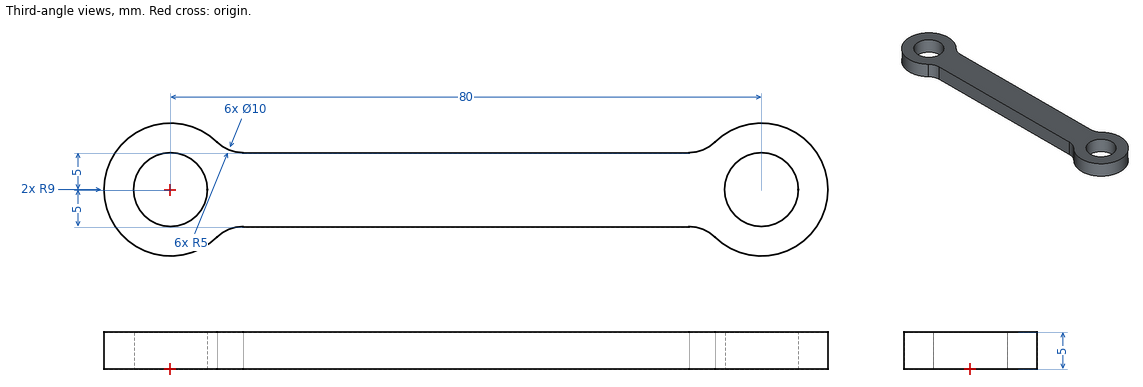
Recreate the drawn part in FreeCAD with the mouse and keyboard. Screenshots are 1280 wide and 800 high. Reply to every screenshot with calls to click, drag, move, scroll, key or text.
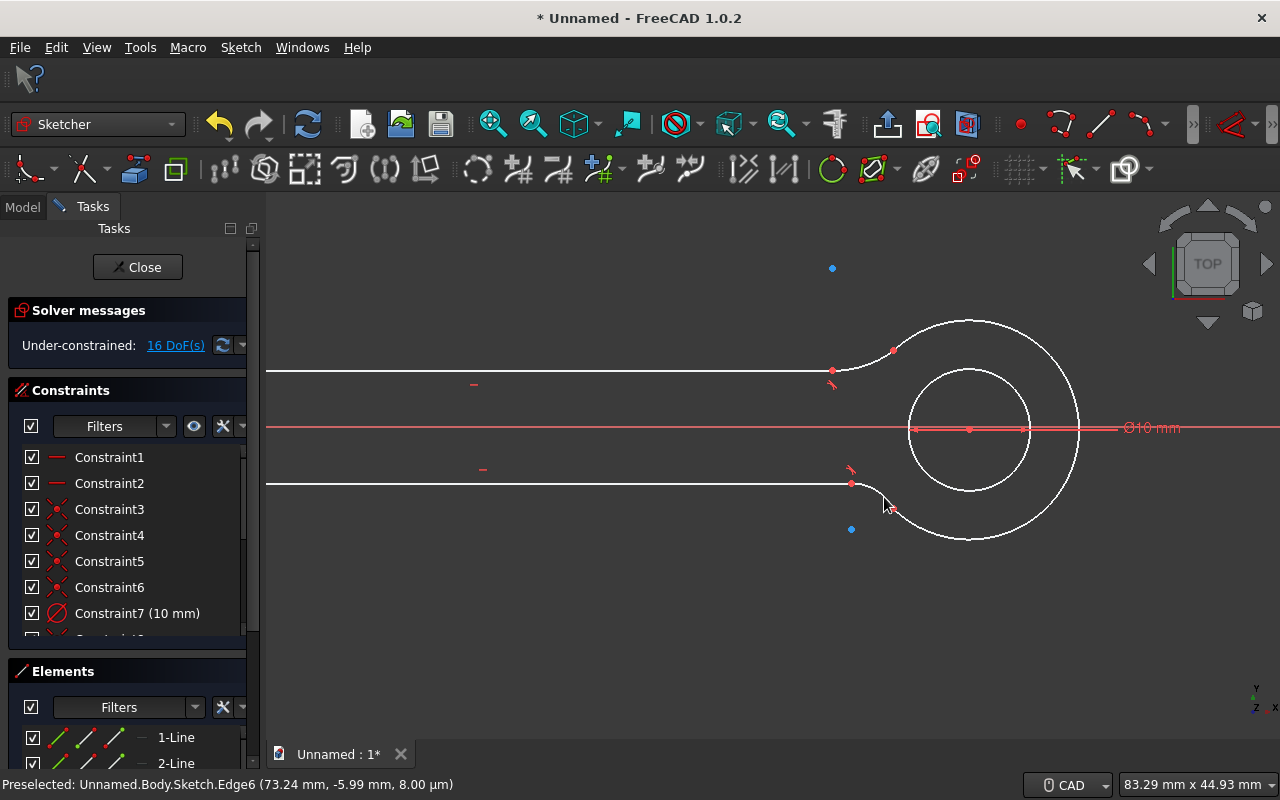
scroll(885, 497, down, 4)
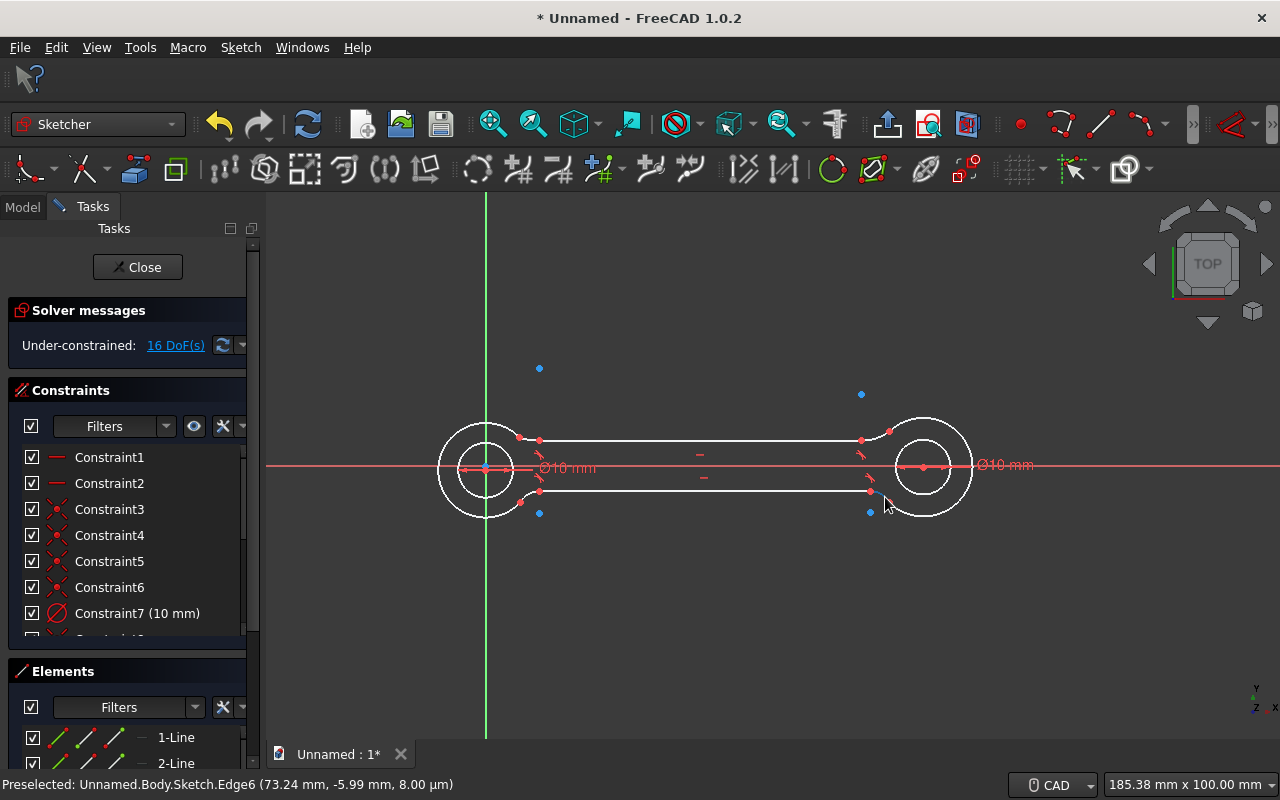
scroll(526, 439, up, 5)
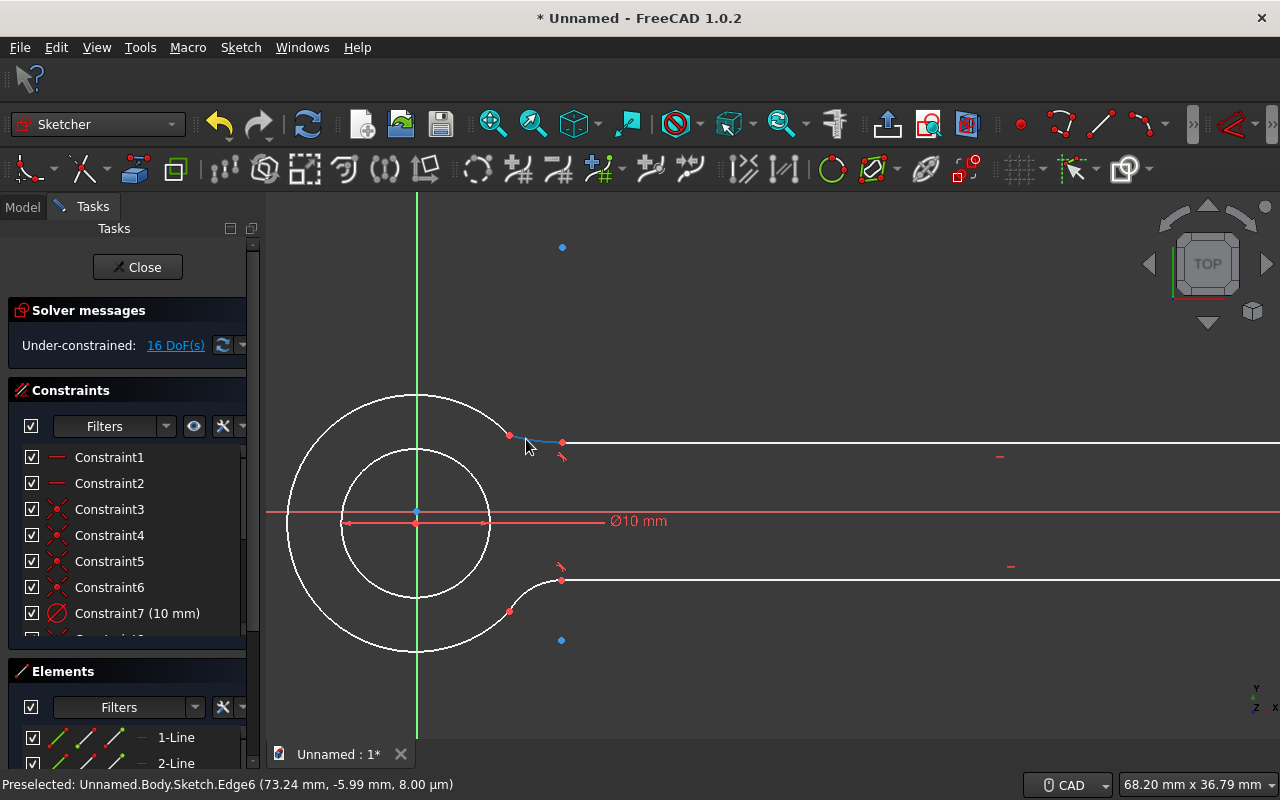
click(525, 439)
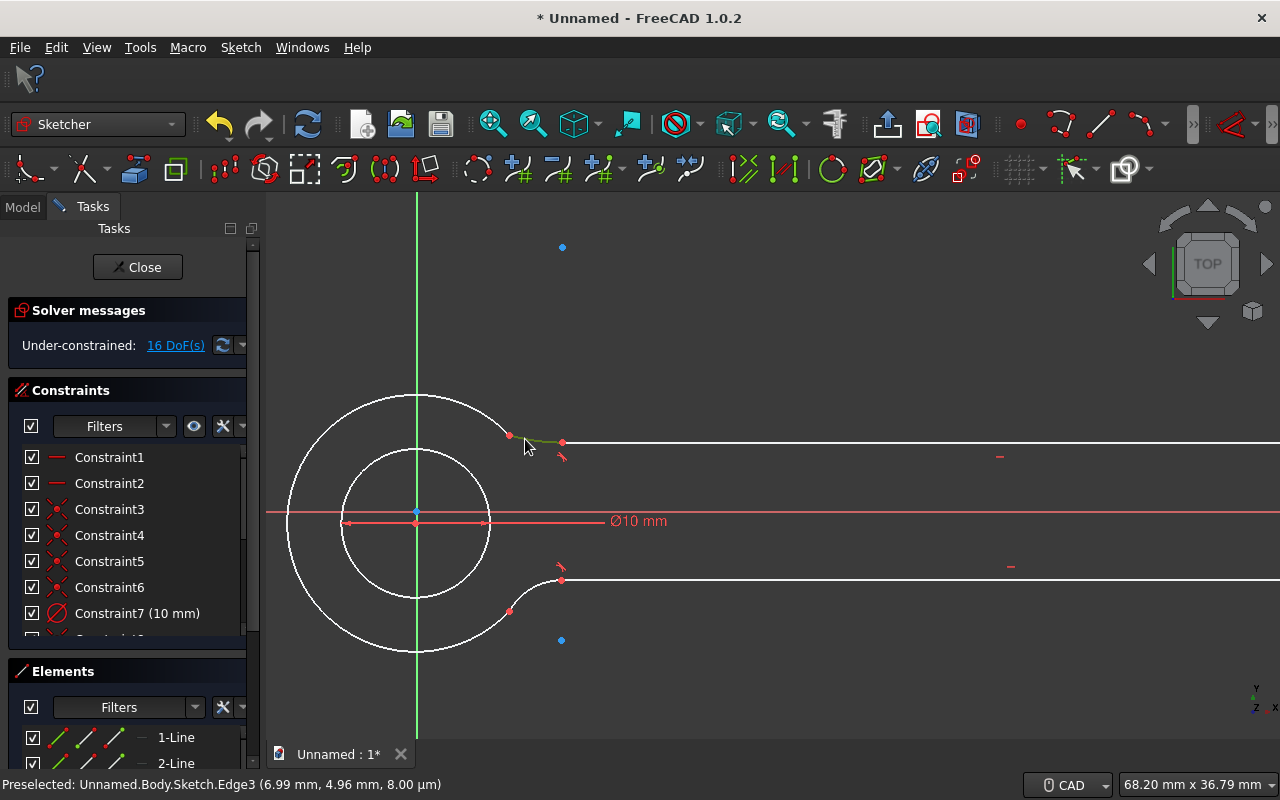
click(341, 419)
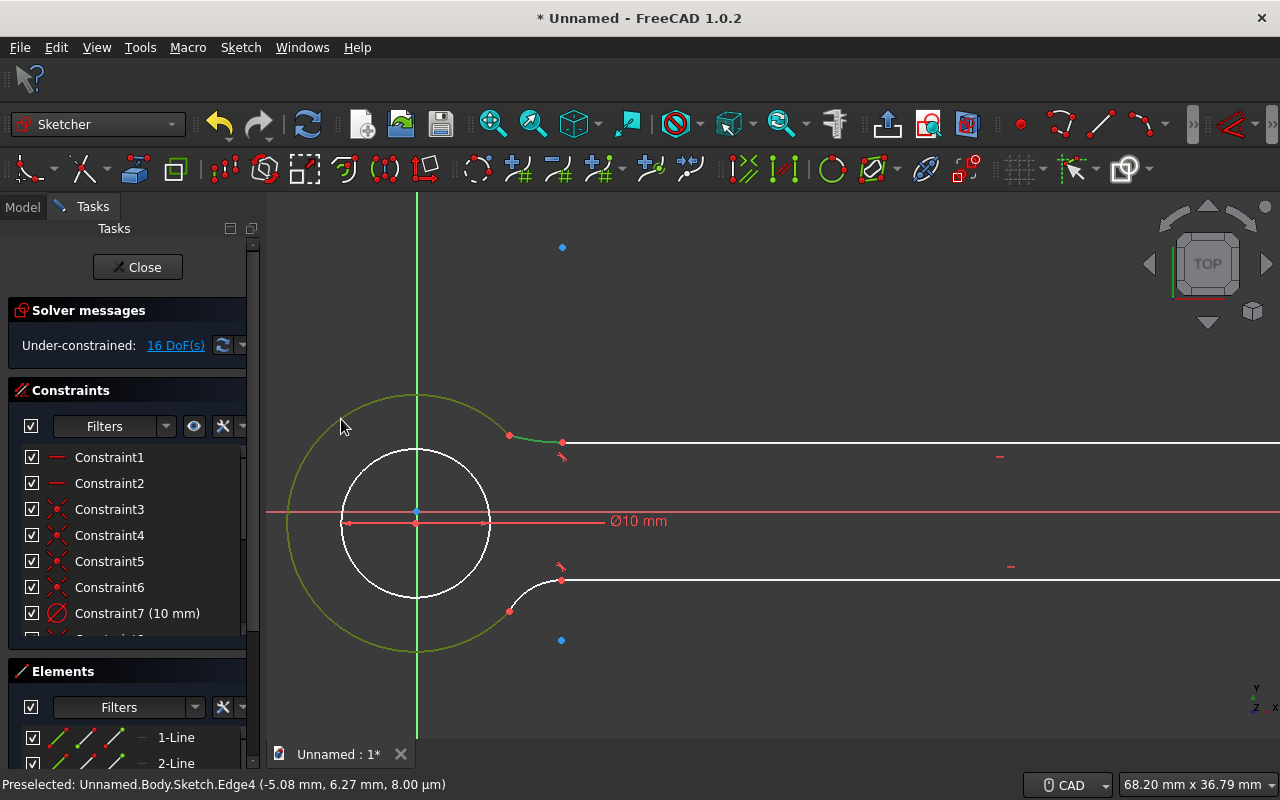
key(t)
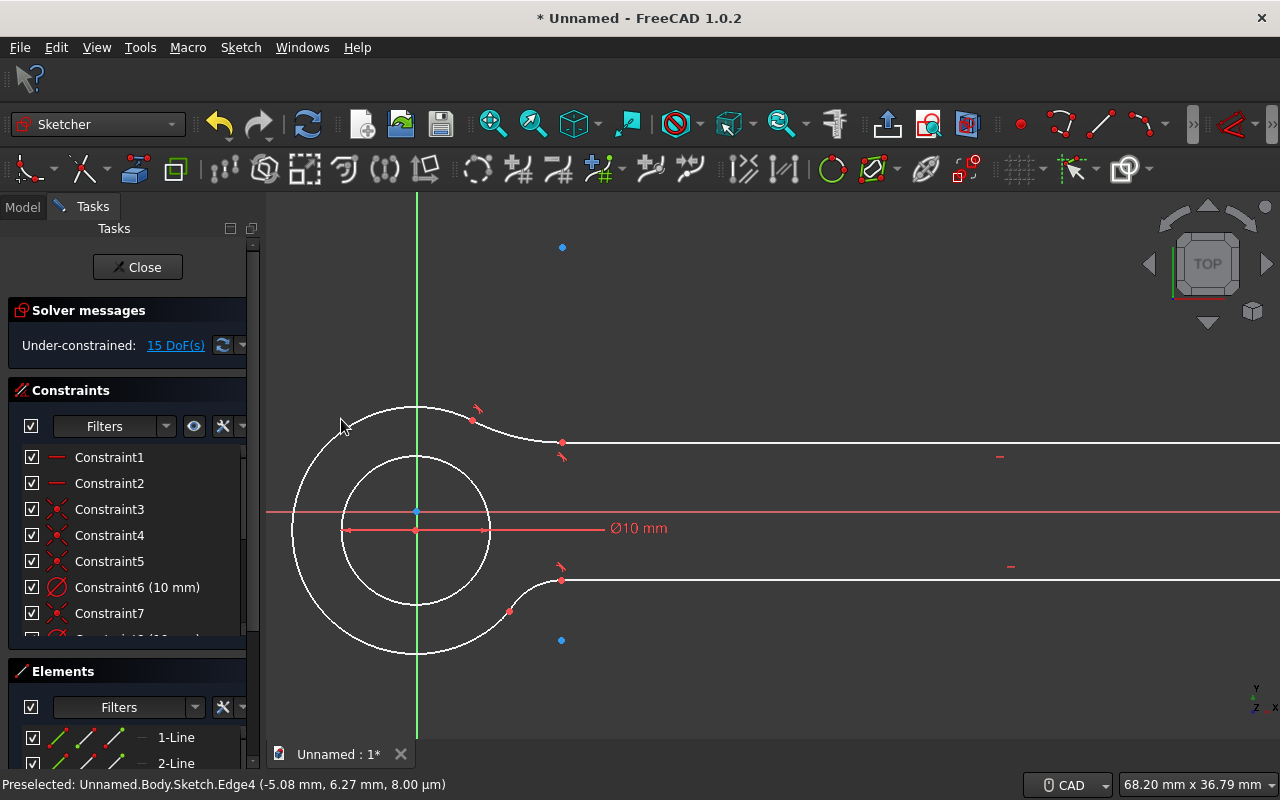
click(322, 450)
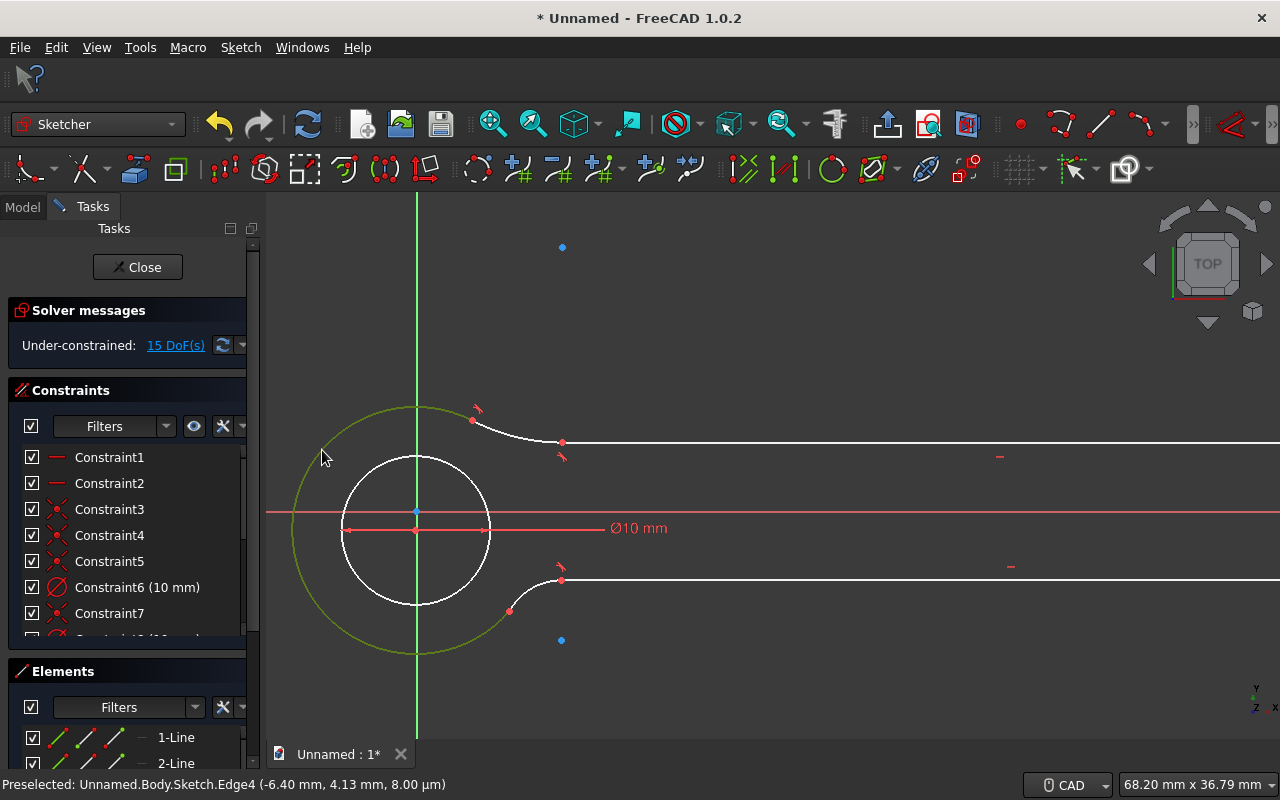
click(543, 583)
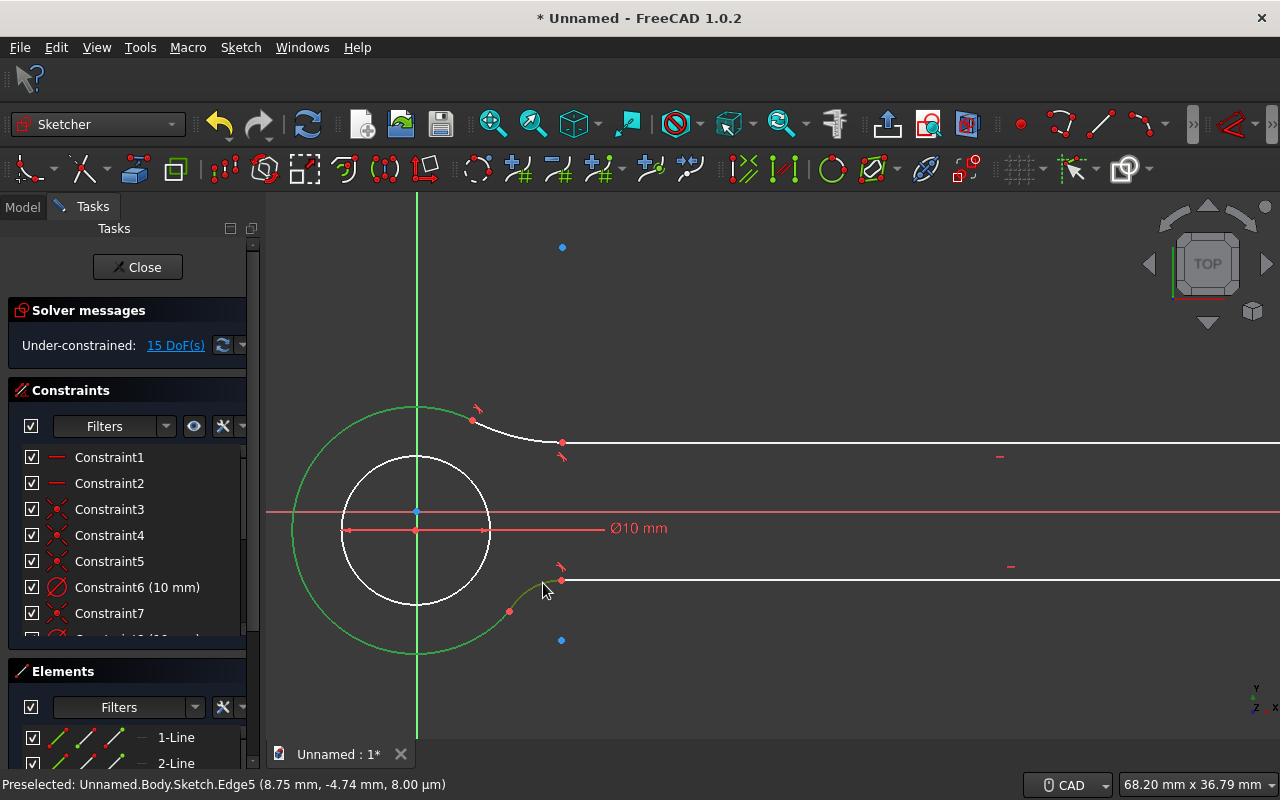
key(t)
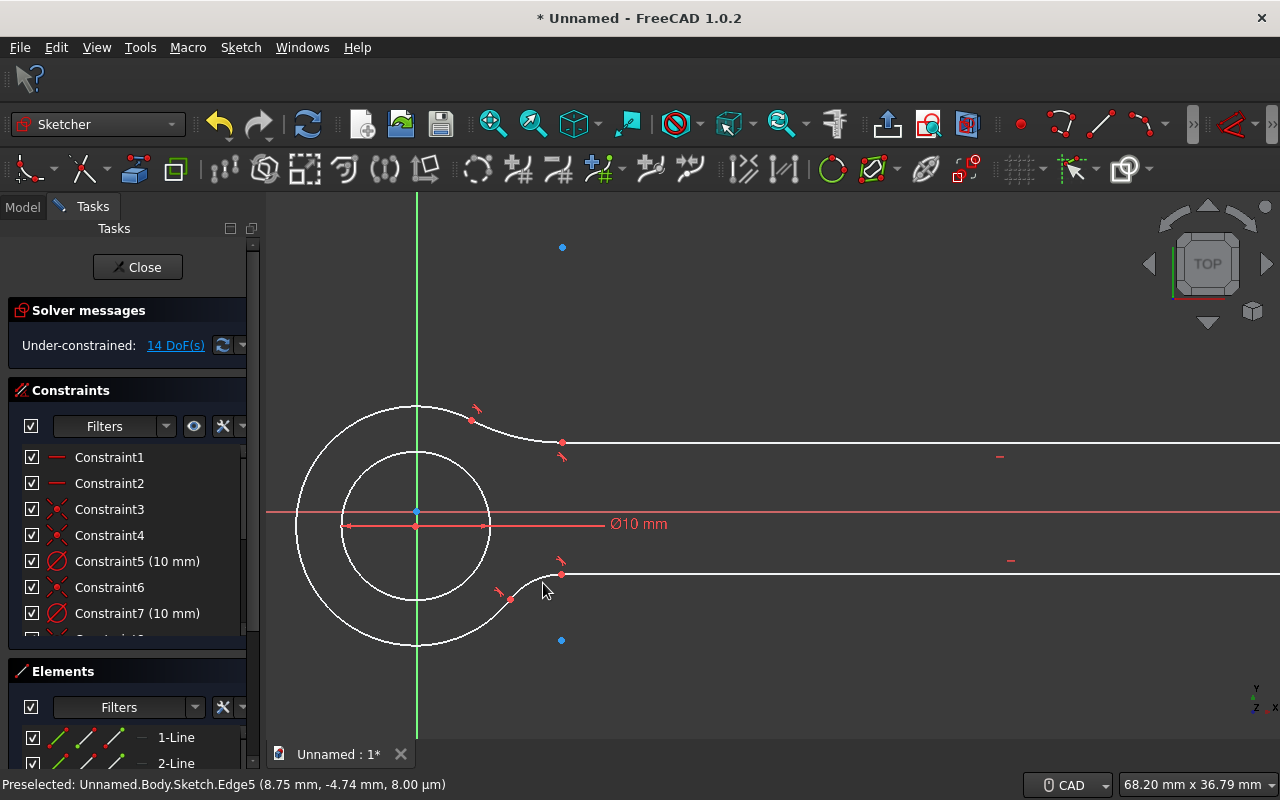
scroll(526, 439, down, 5)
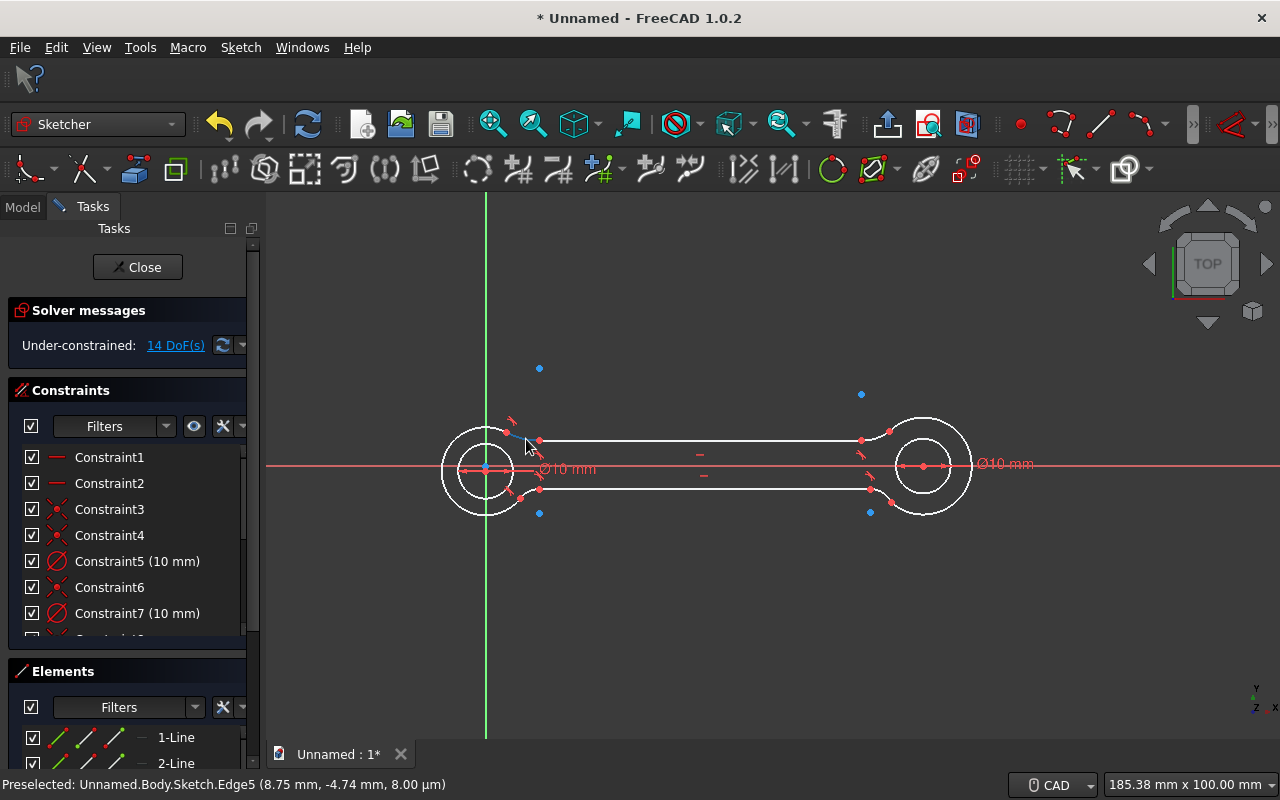
scroll(887, 496, up, 3)